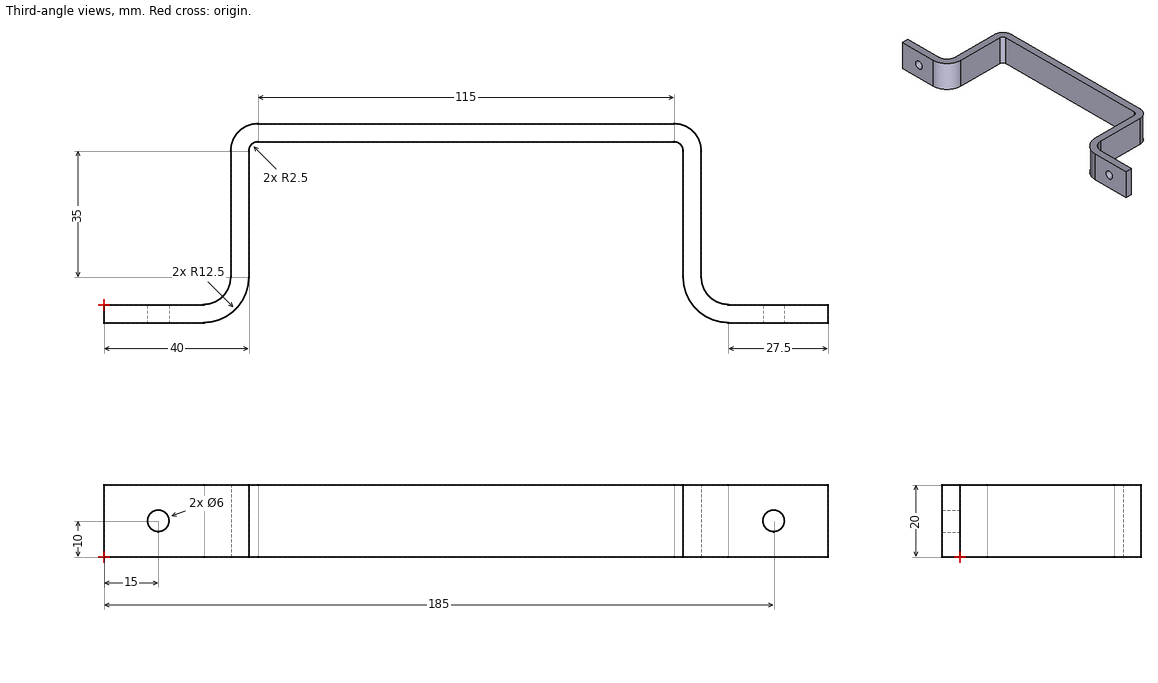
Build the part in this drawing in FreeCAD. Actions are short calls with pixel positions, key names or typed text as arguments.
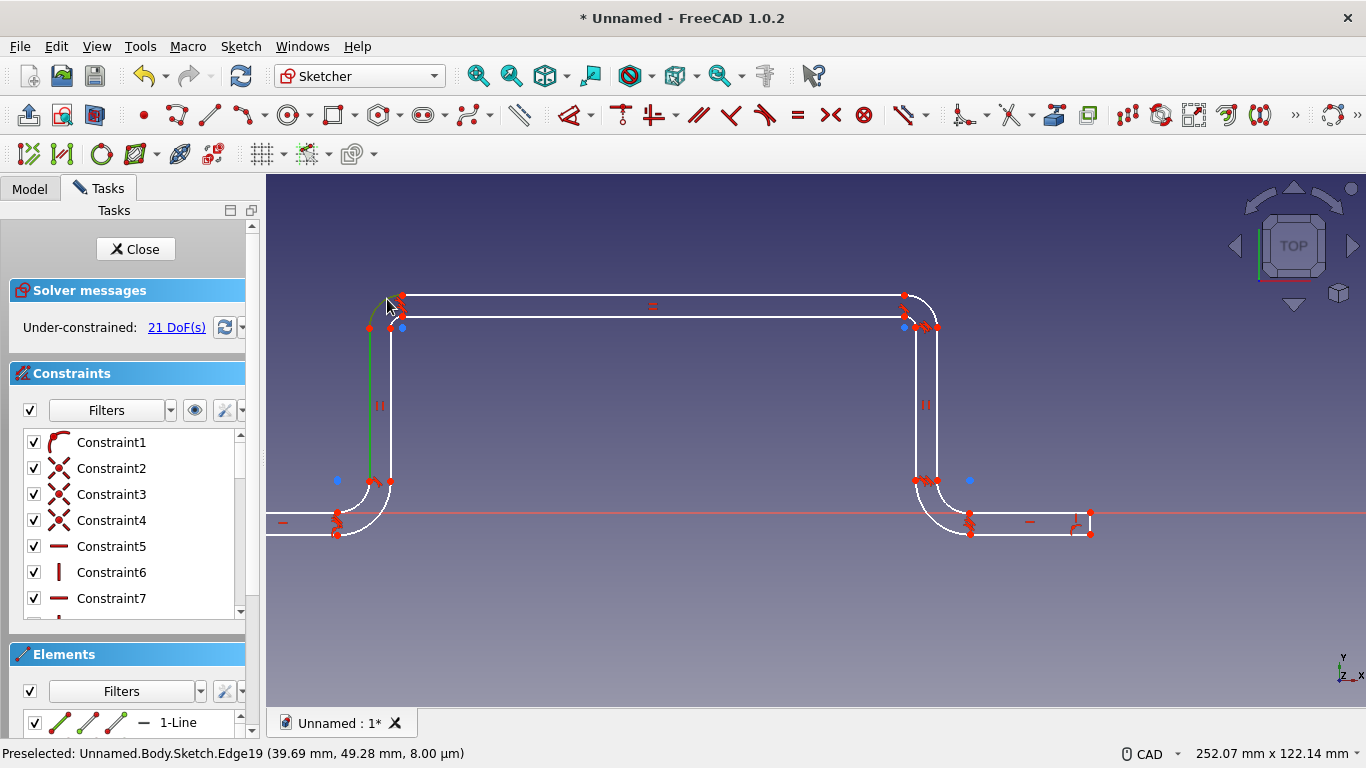
click(765, 116)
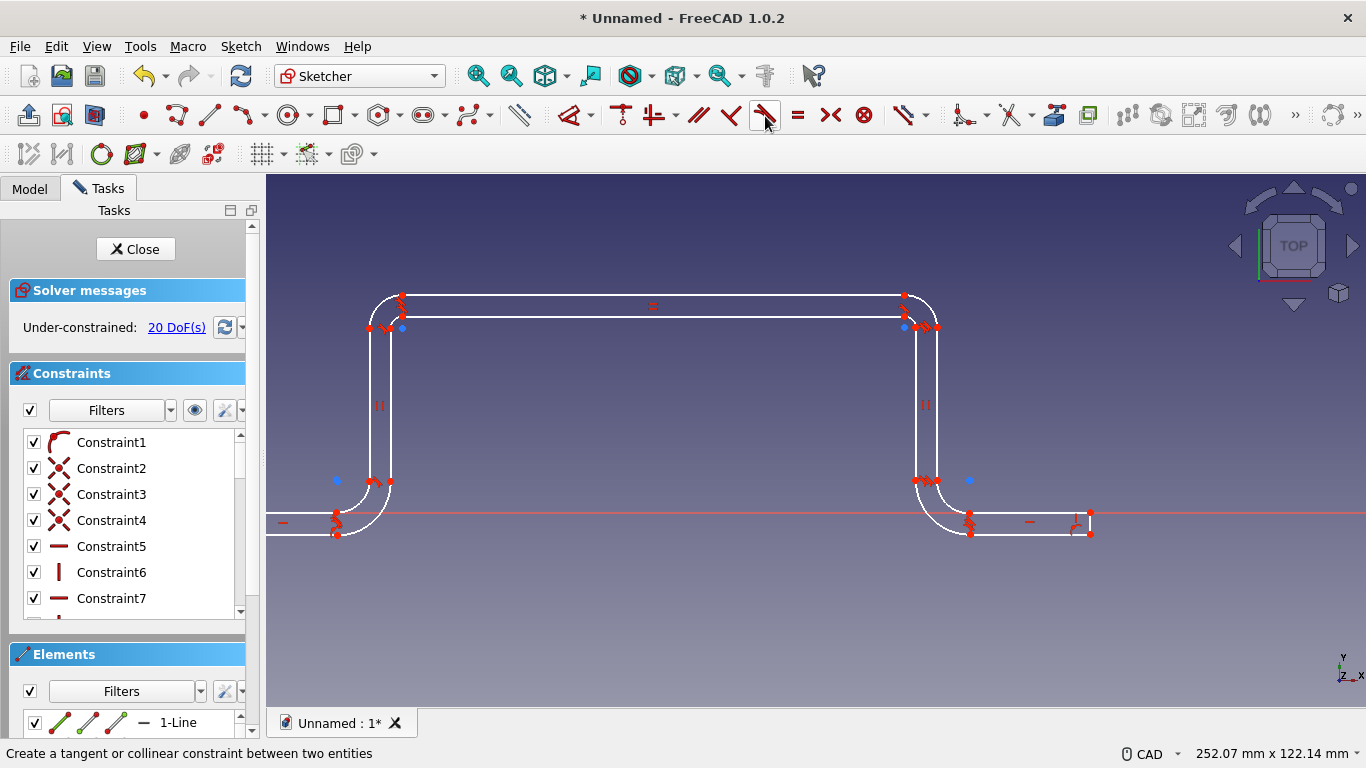
click(370, 374)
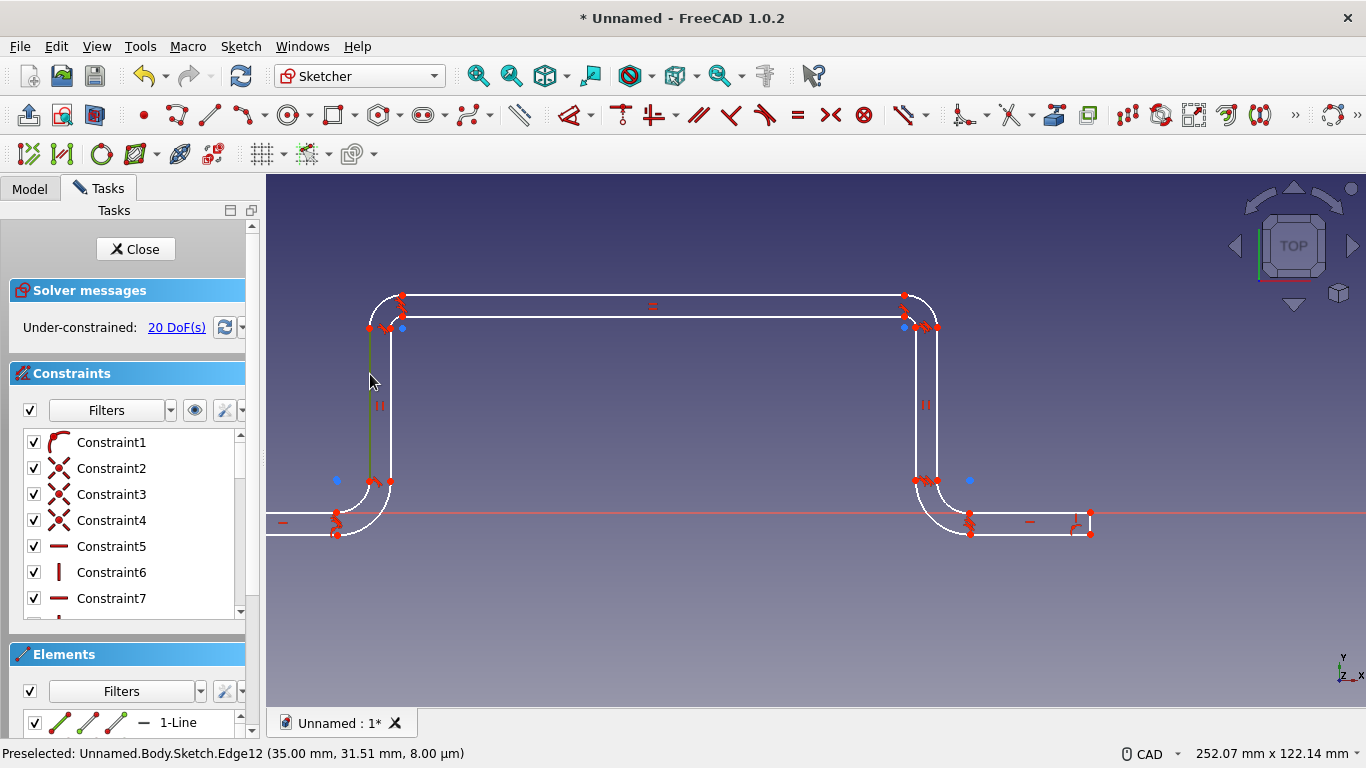
click(351, 509)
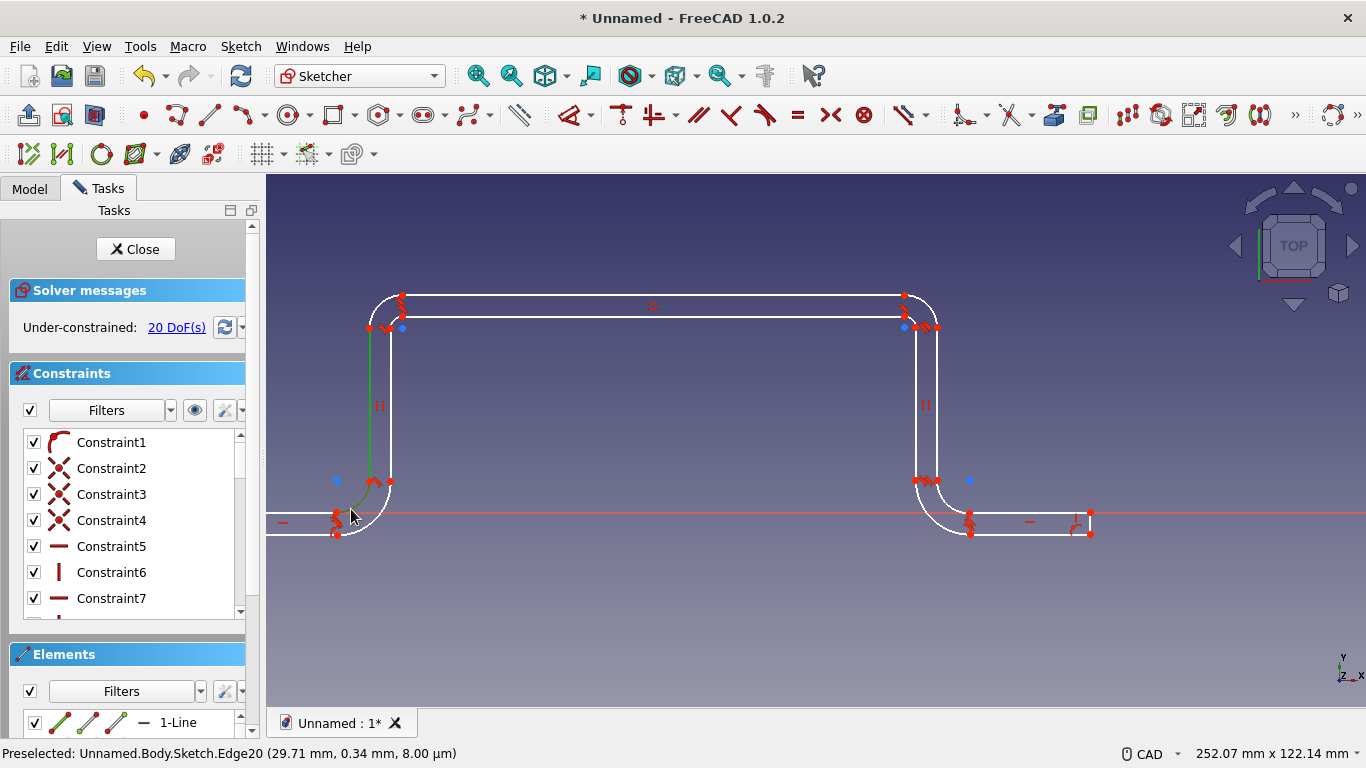
click(765, 116)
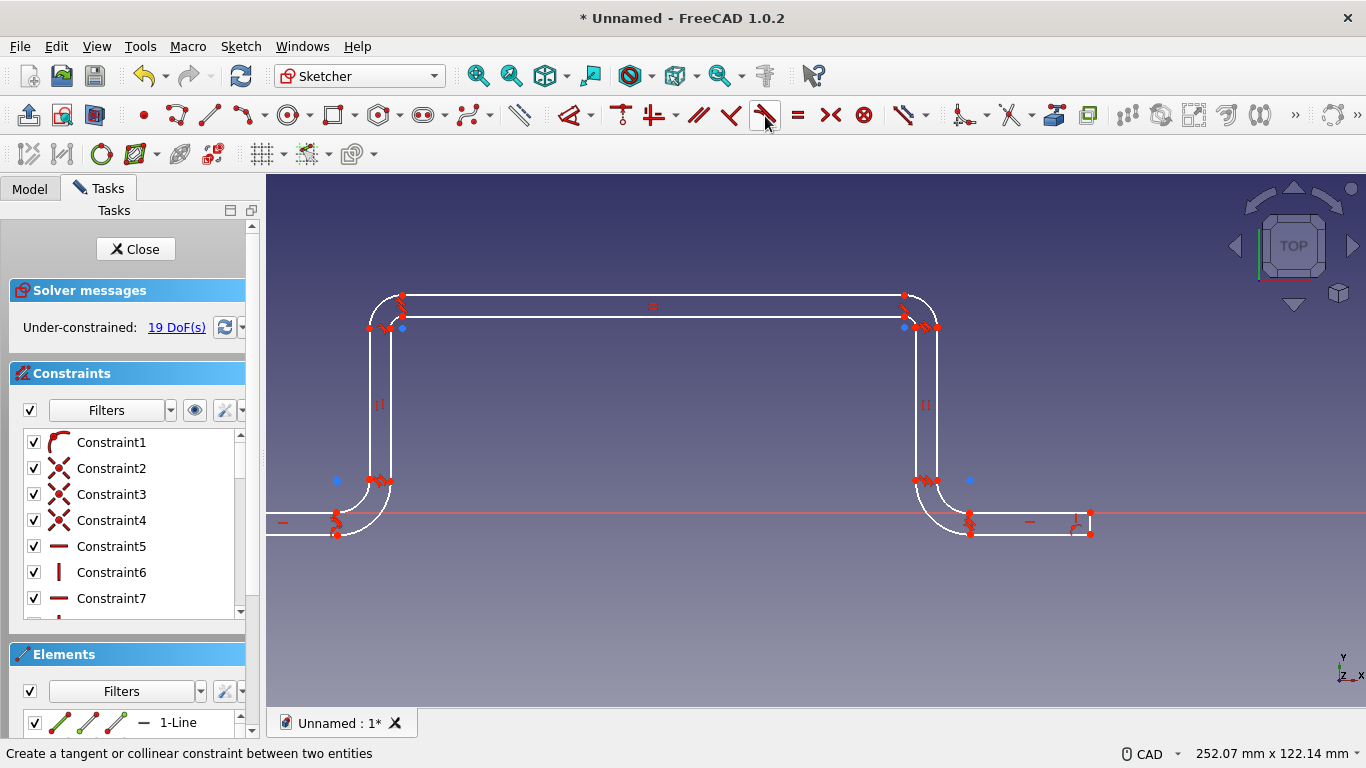
scroll(939, 494, down, 2)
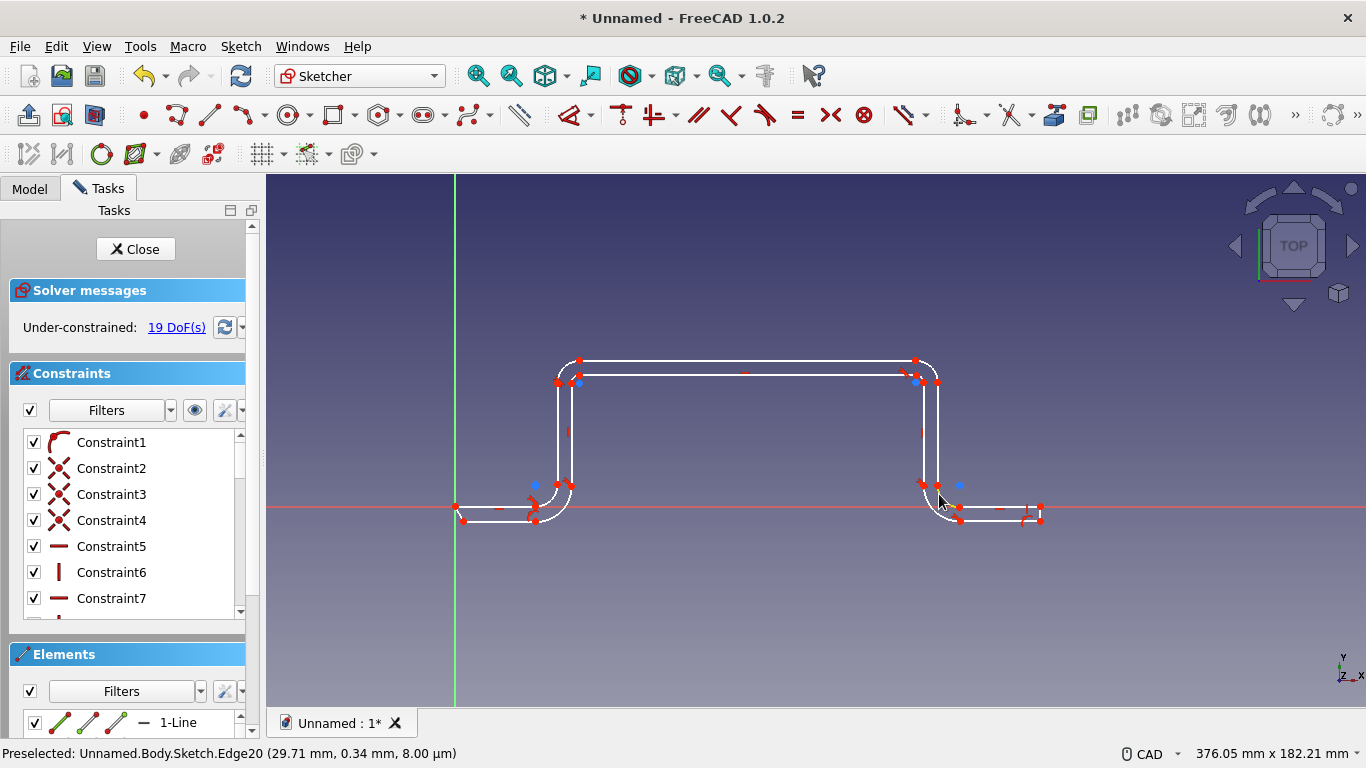
scroll(461, 517, up, 5)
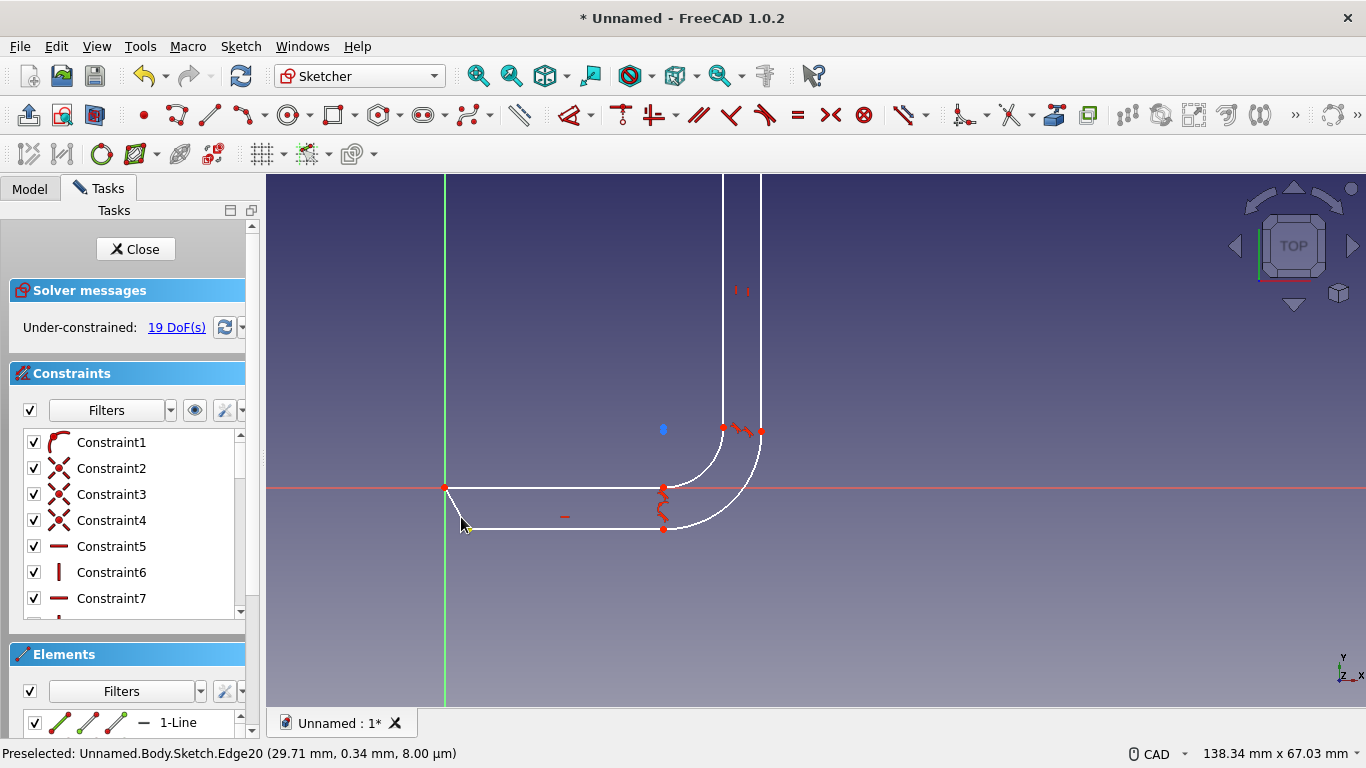
click(461, 517)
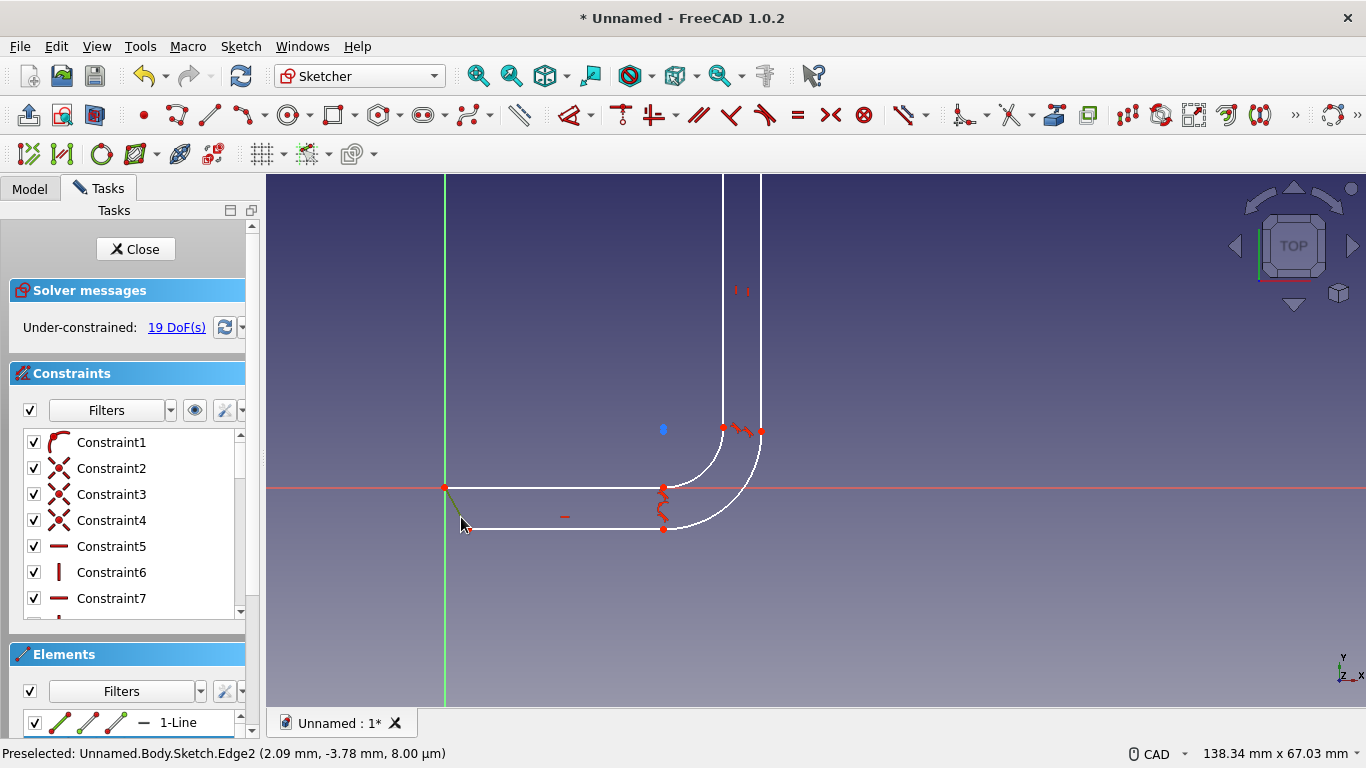
key(v)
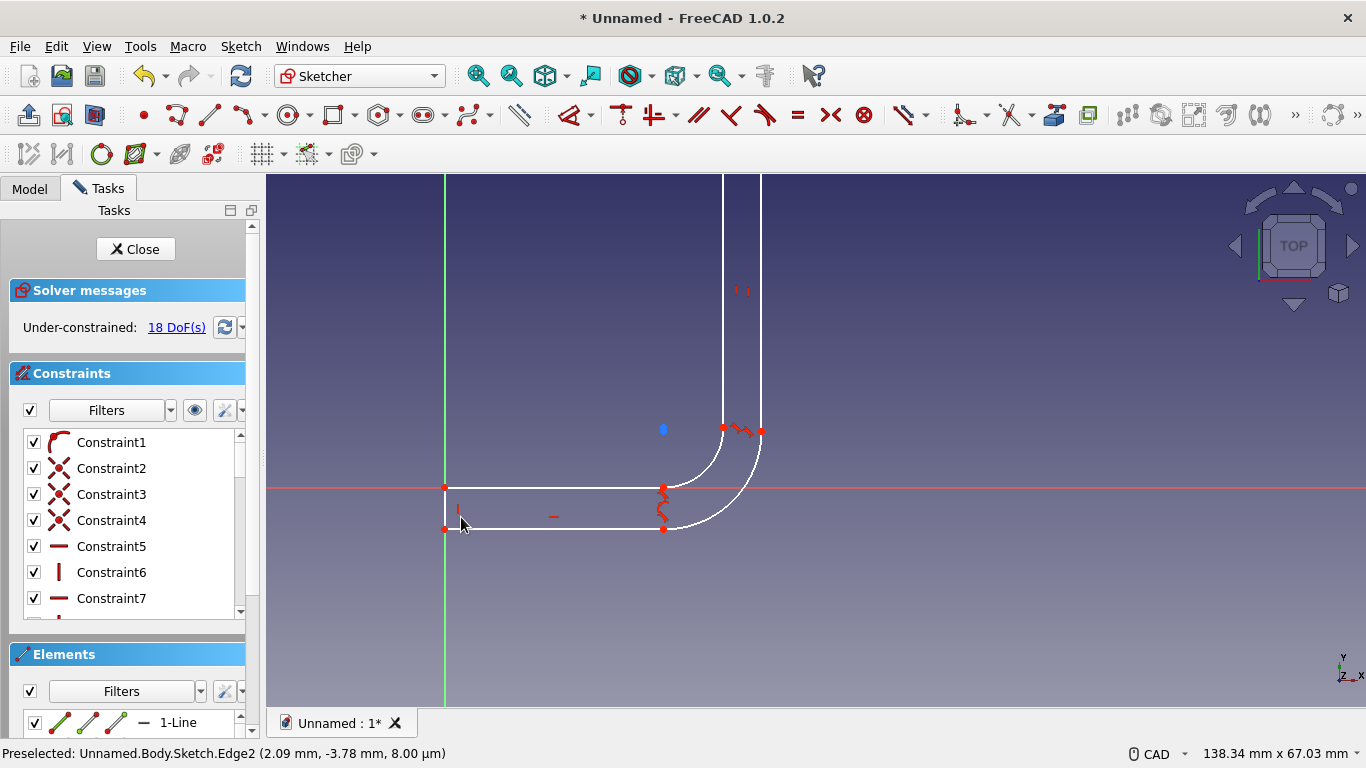
scroll(461, 517, down, 5)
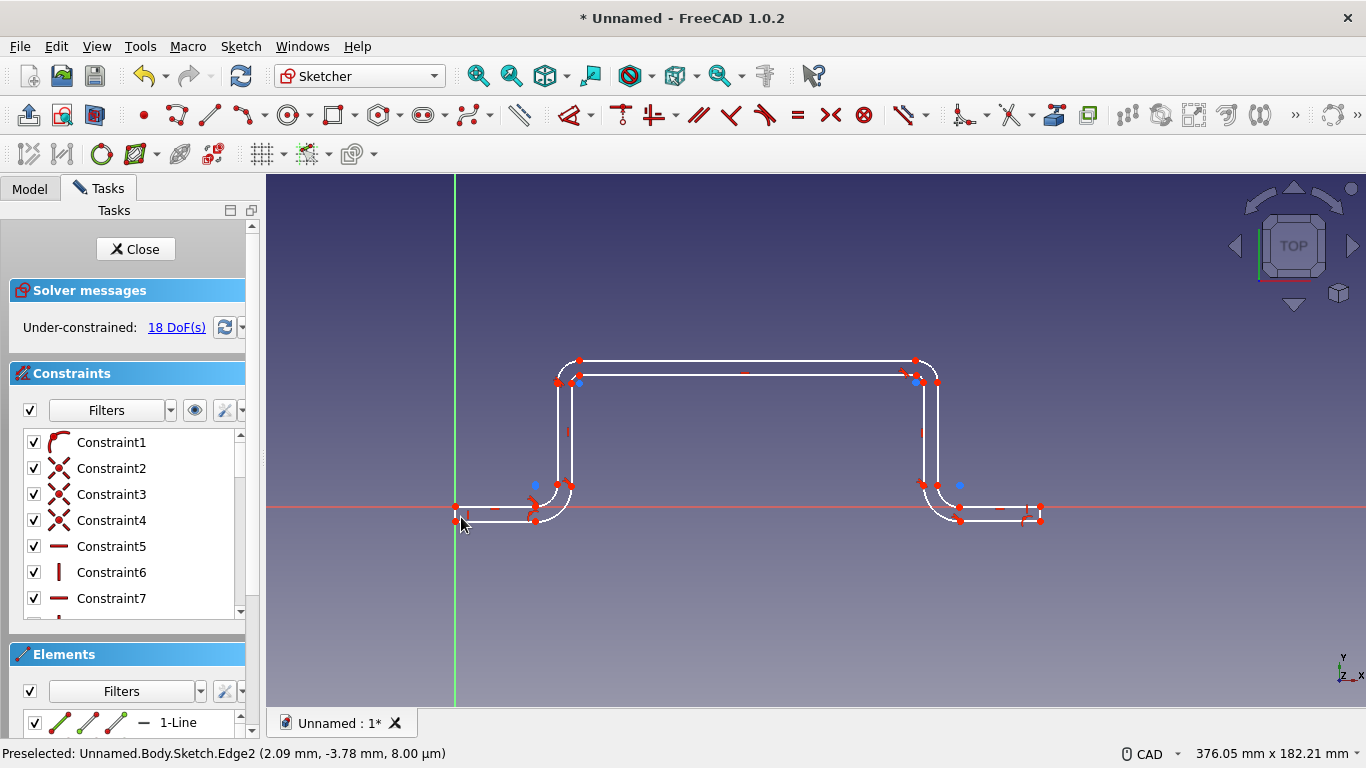
click(1016, 507)